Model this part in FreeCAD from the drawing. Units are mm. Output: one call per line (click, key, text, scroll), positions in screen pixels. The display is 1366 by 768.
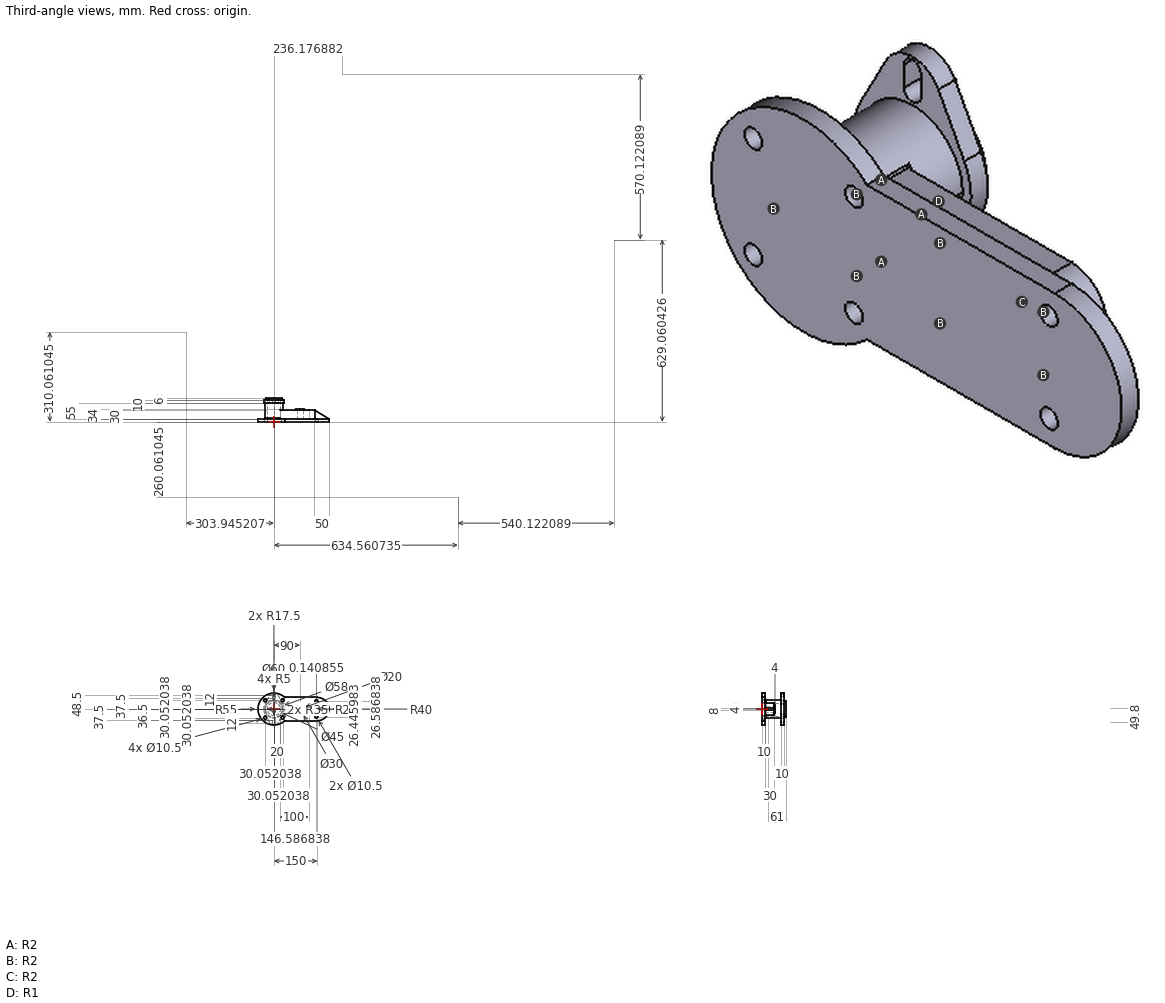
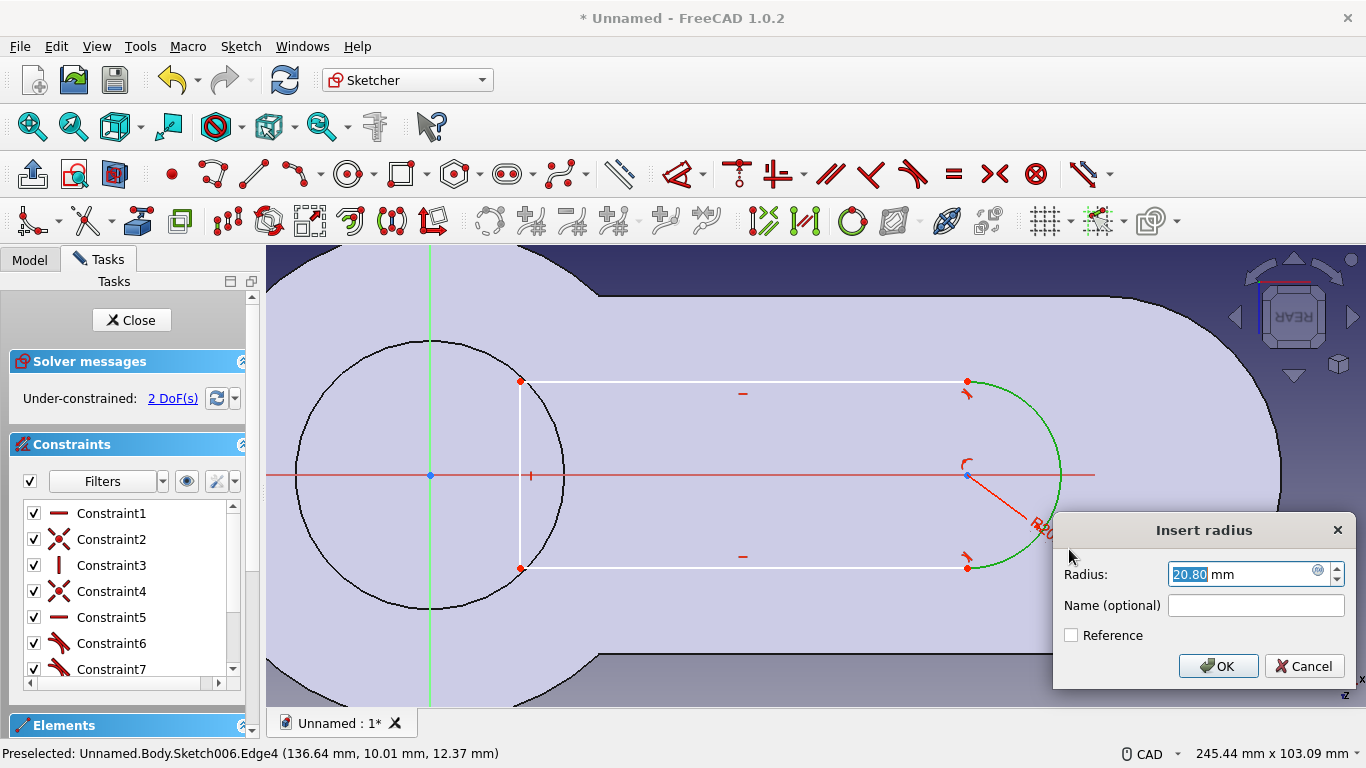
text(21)
key(Return)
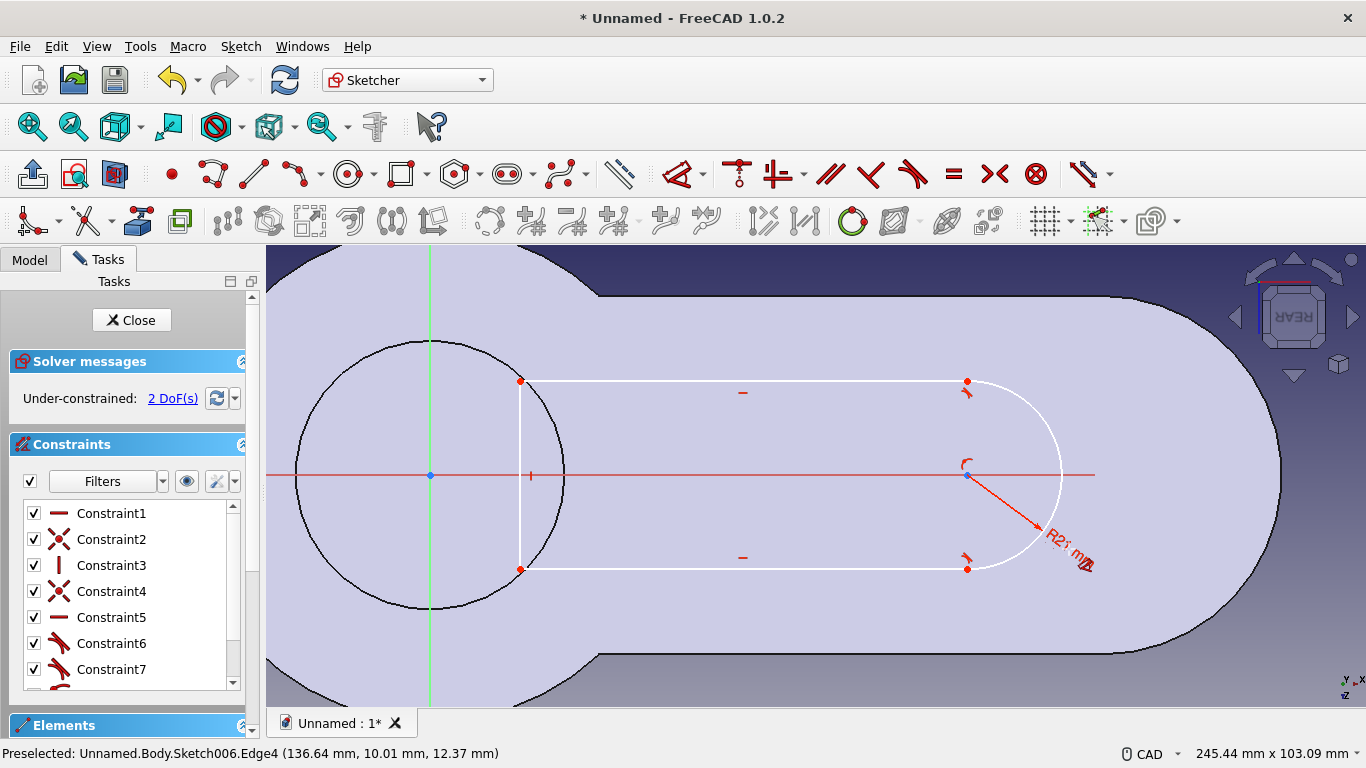
click(833, 381)
click(744, 347)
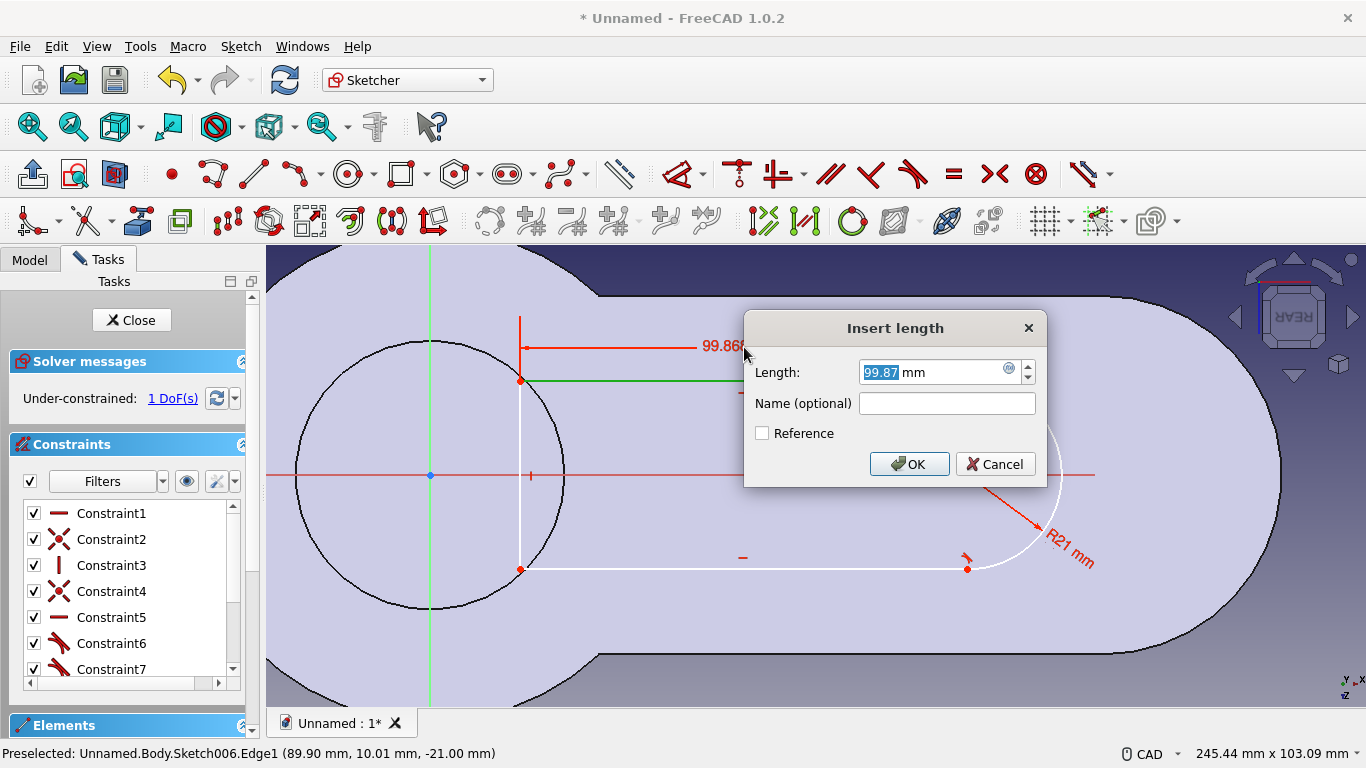
text(100)
key(Return)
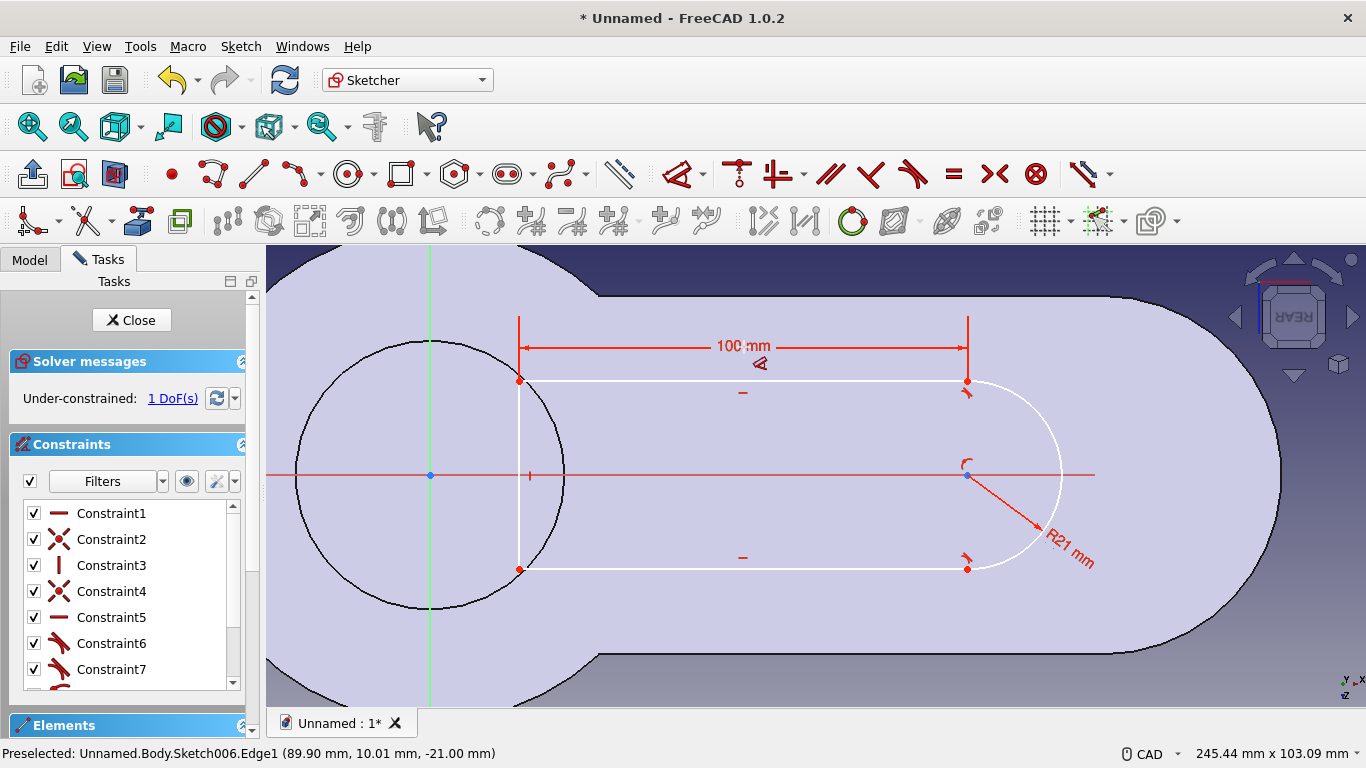
click(519, 381)
click(475, 347)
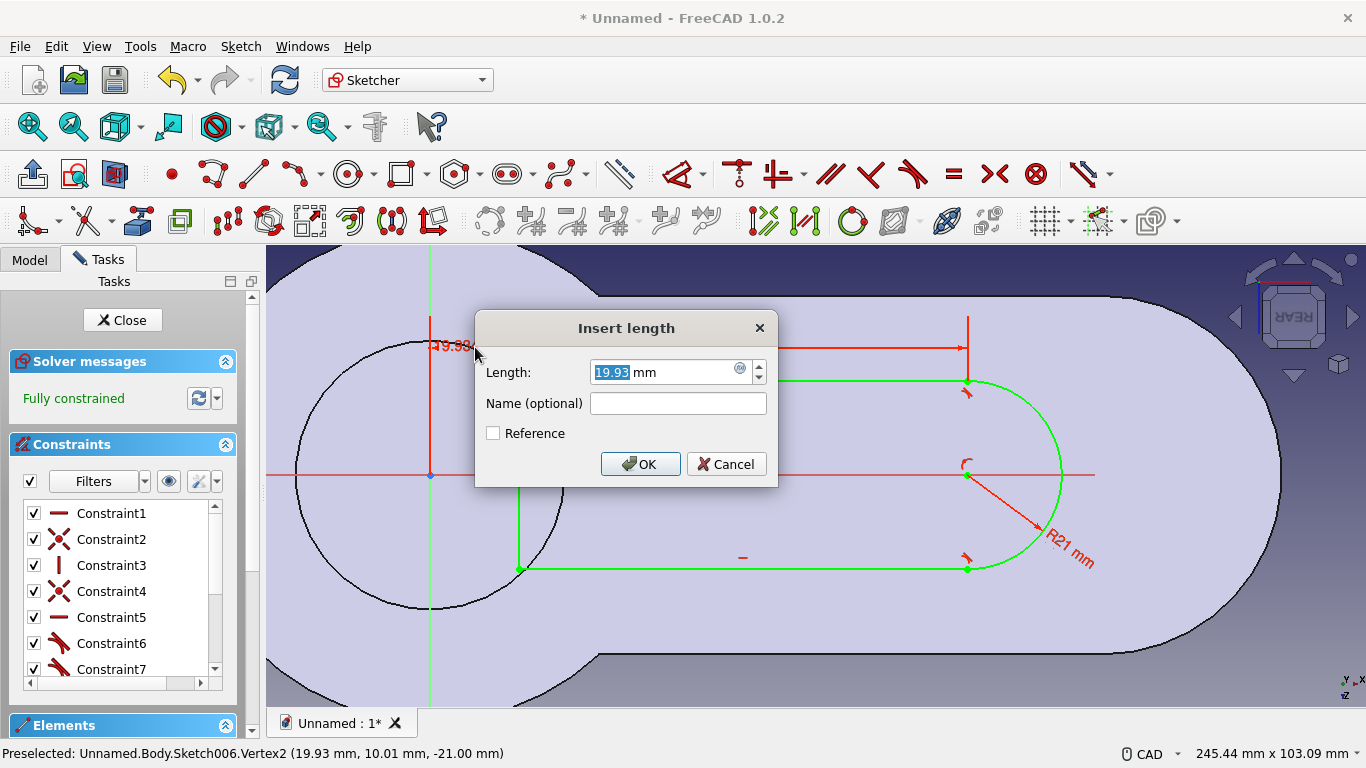
text(20)
key(Return)
key(Escape)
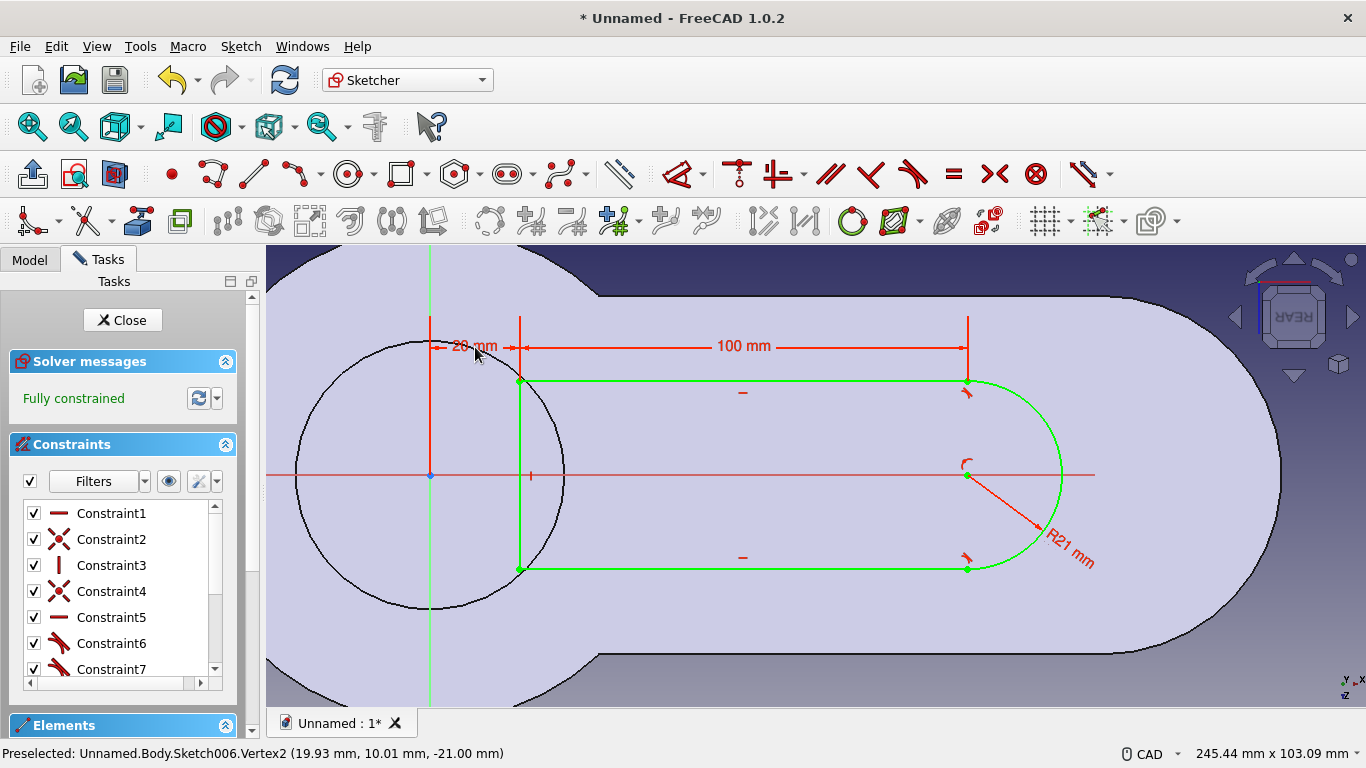
click(123, 320)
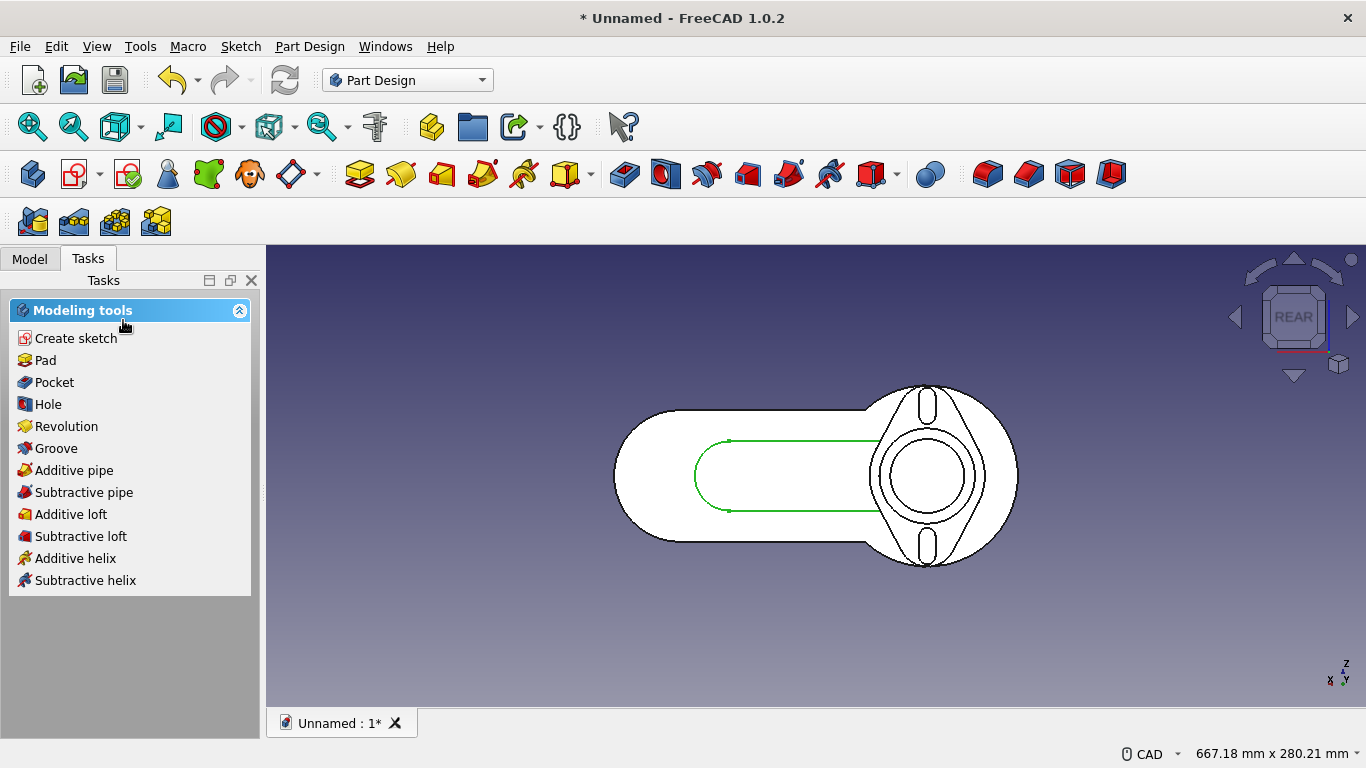
click(360, 174)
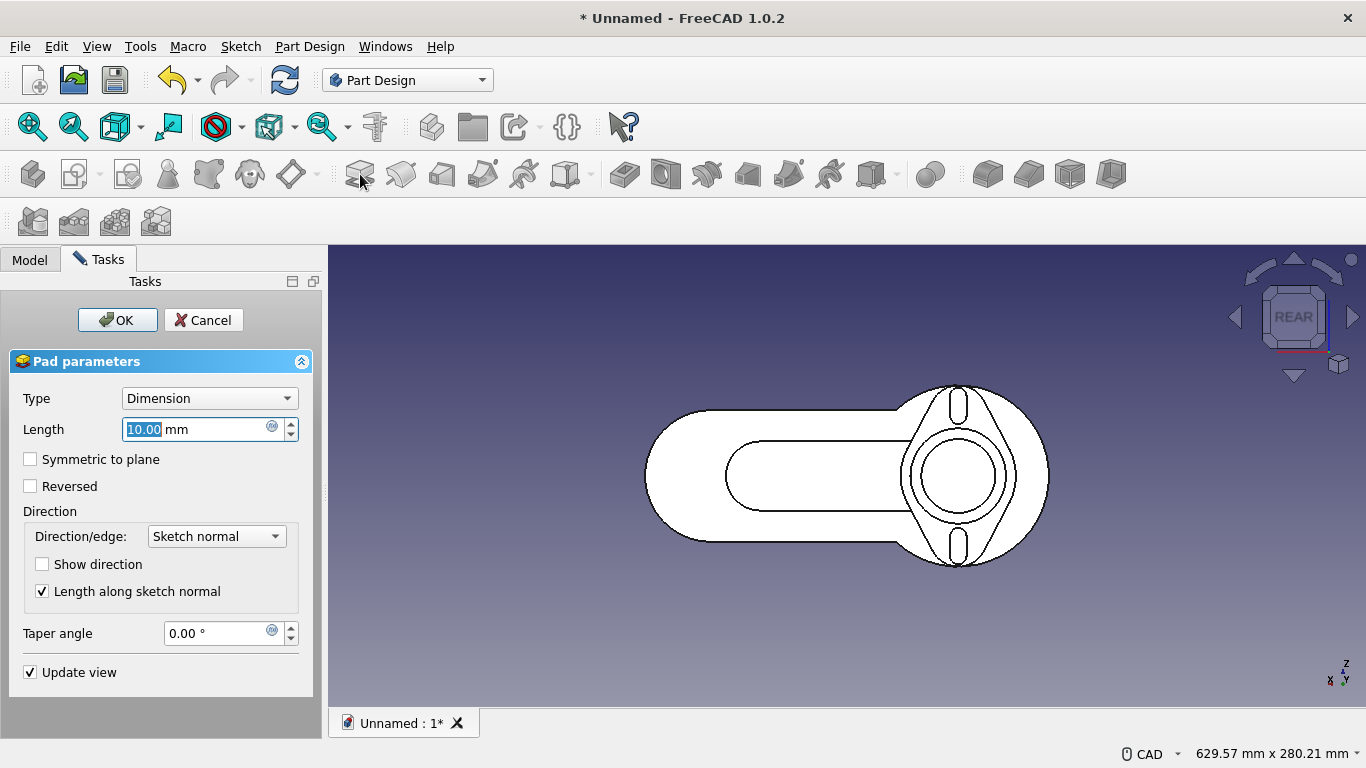
text(30)
key(Tab)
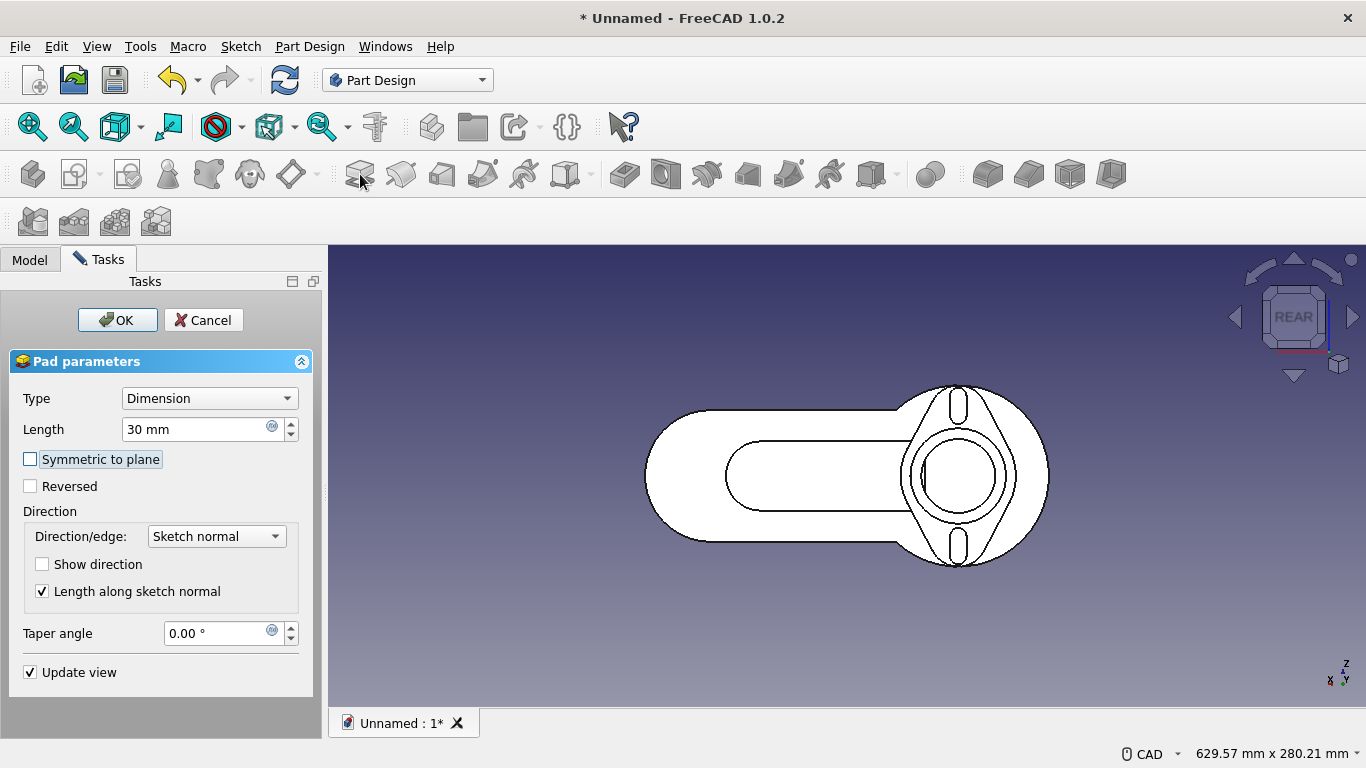
click(118, 320)